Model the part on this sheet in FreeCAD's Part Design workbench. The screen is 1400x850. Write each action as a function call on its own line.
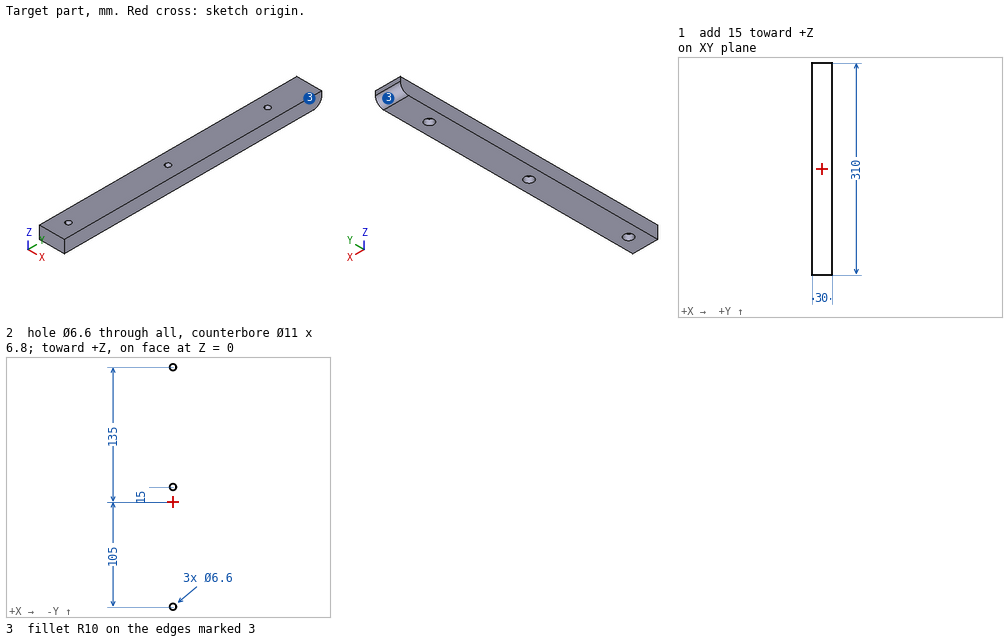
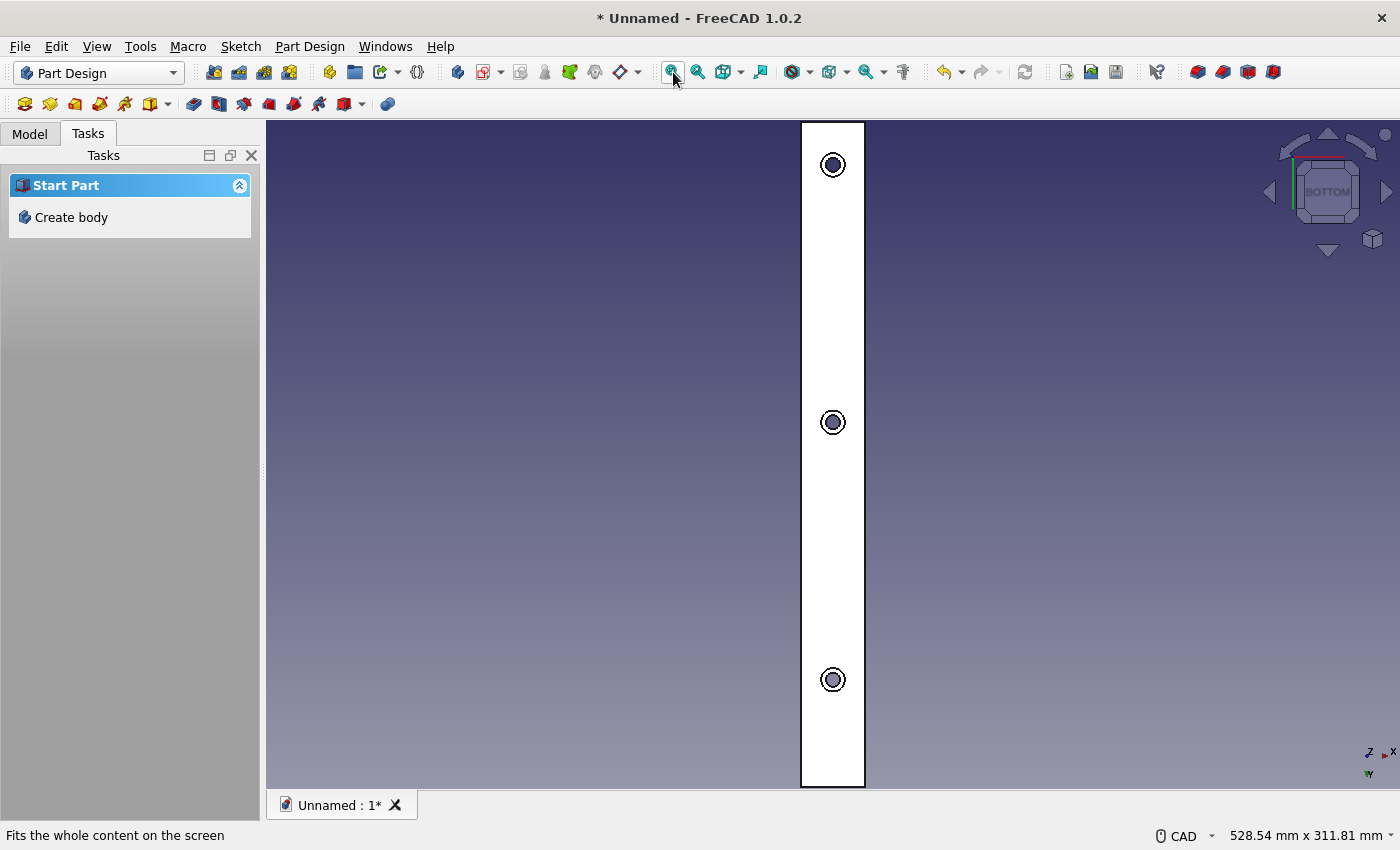
key(4)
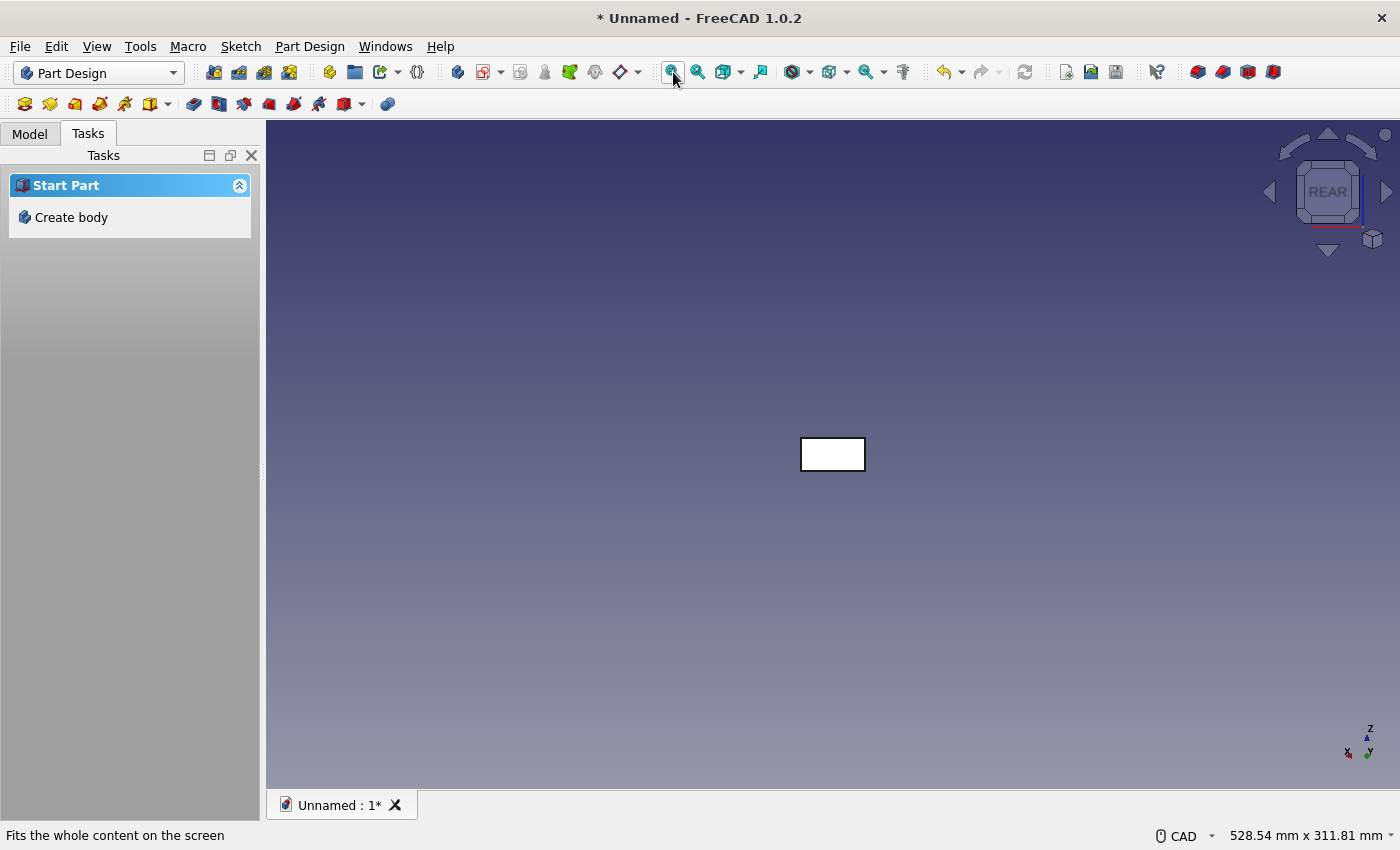
click(673, 72)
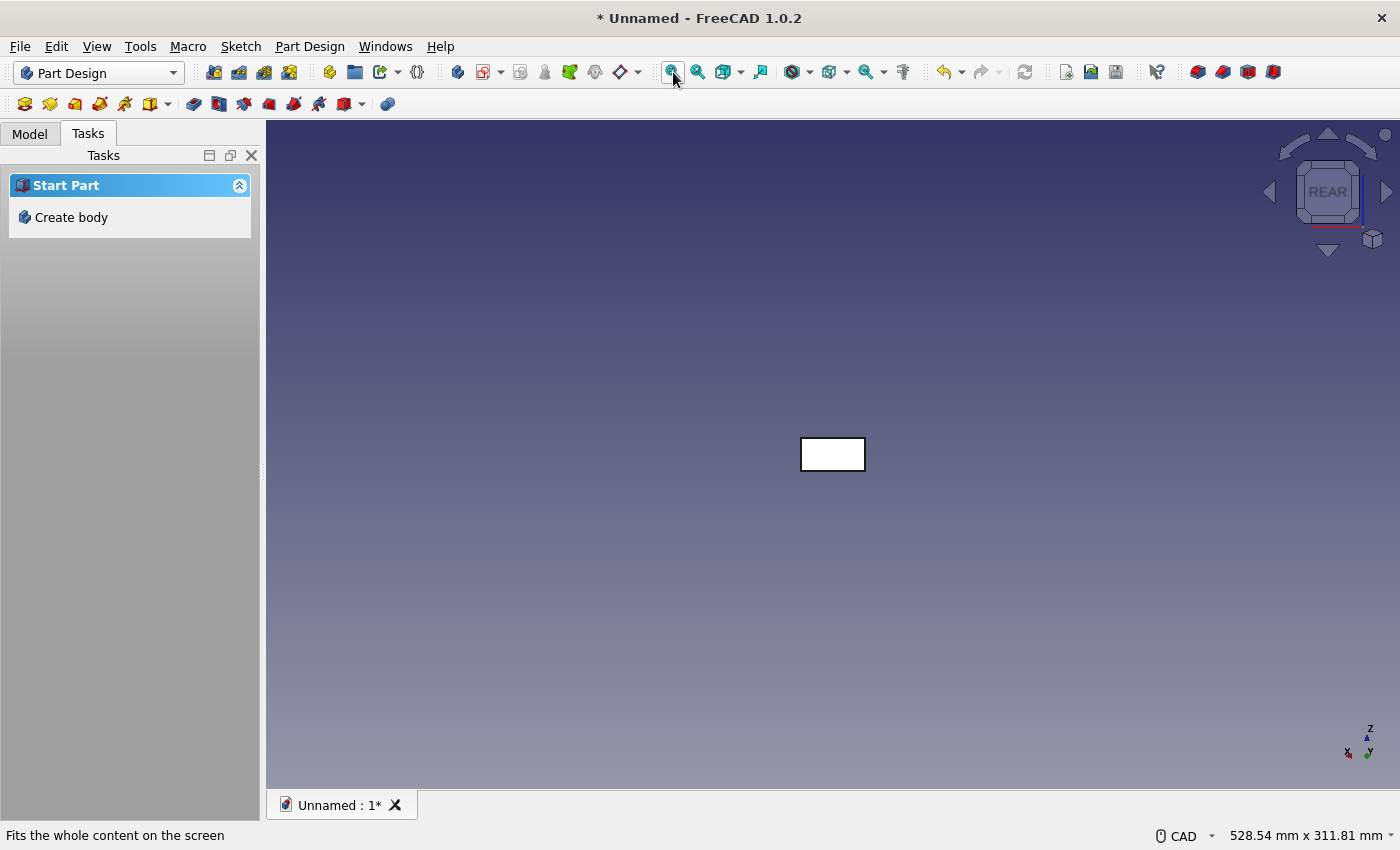
click(833, 470)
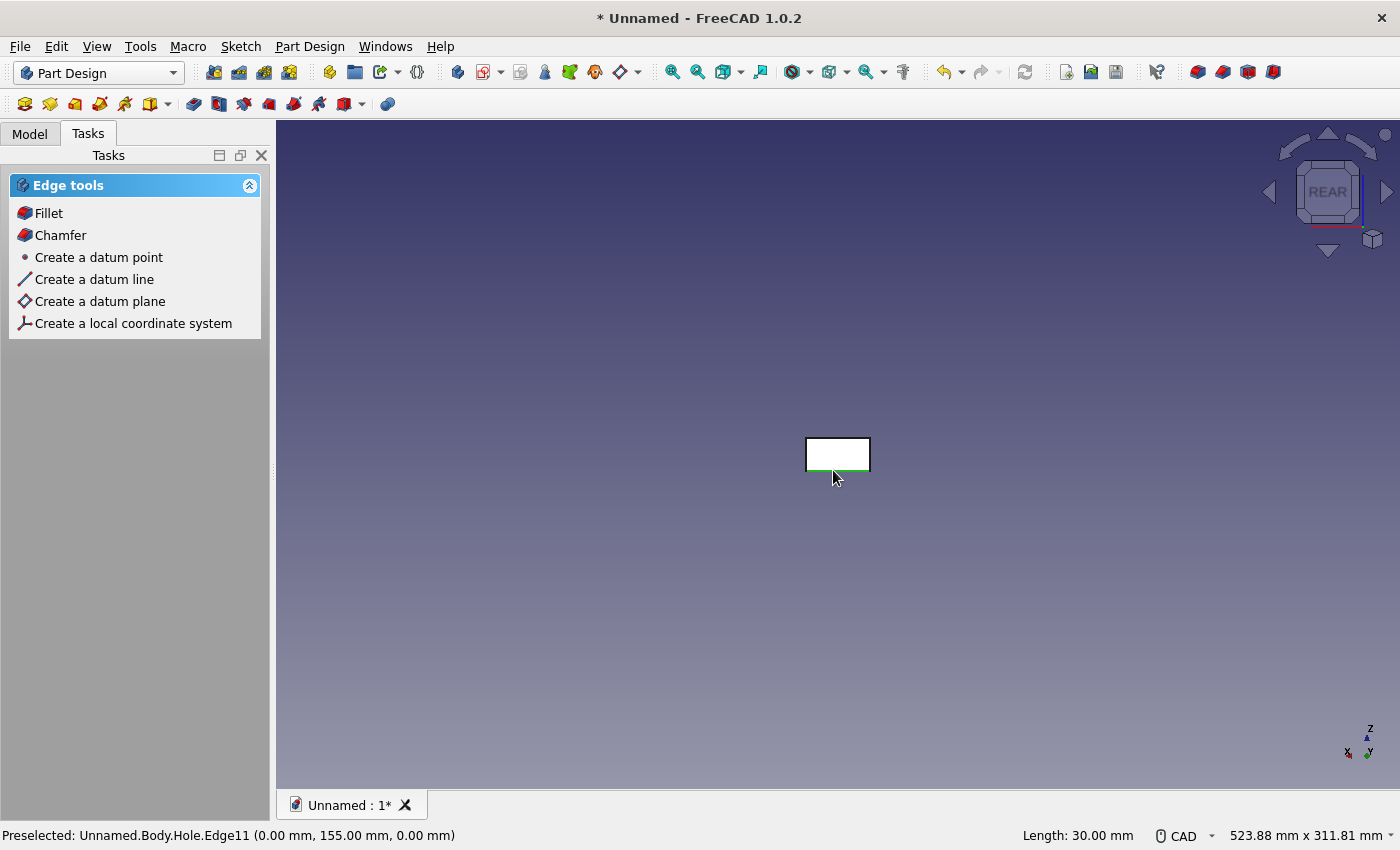
click(1198, 72)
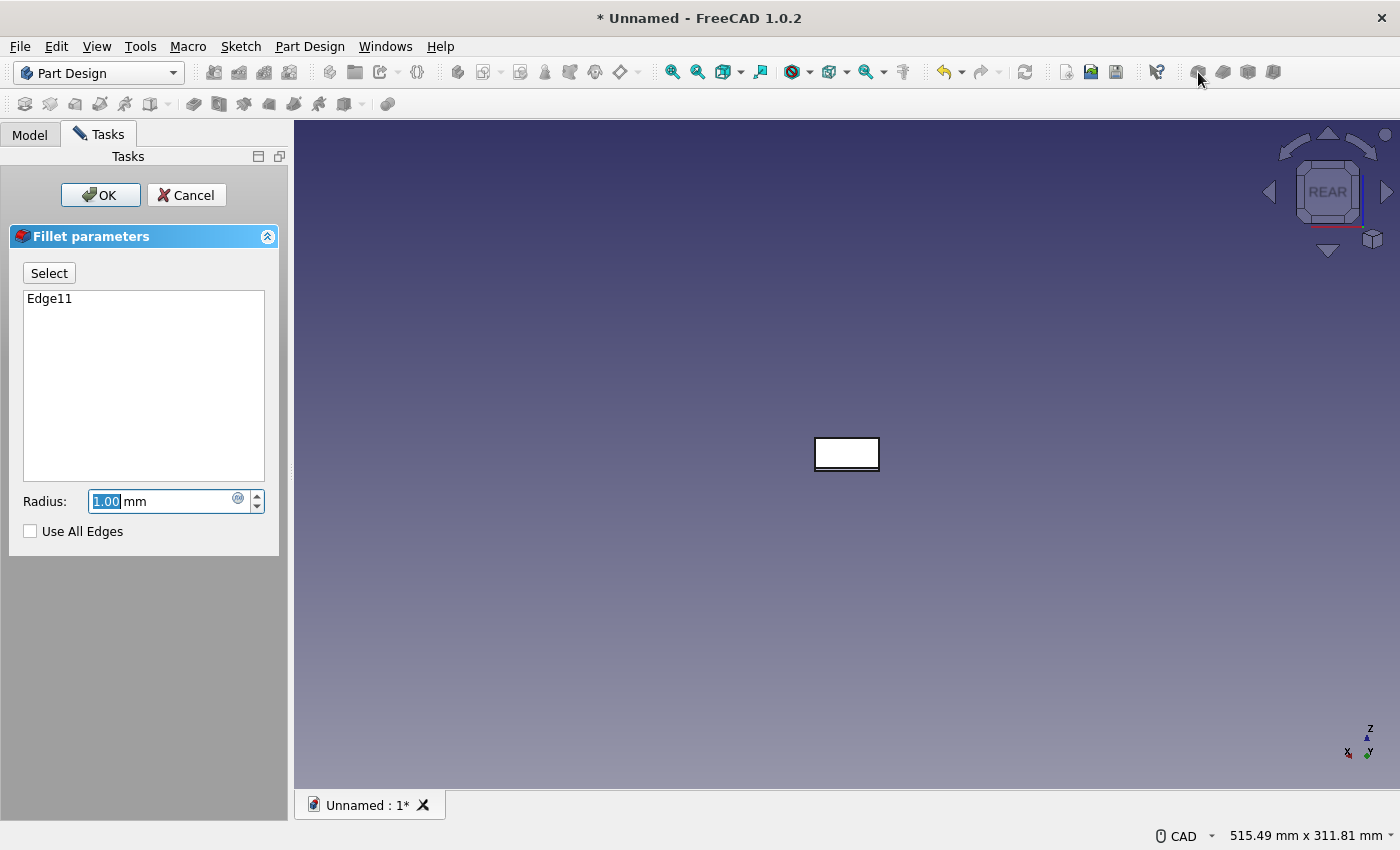
text(10)
key(Tab)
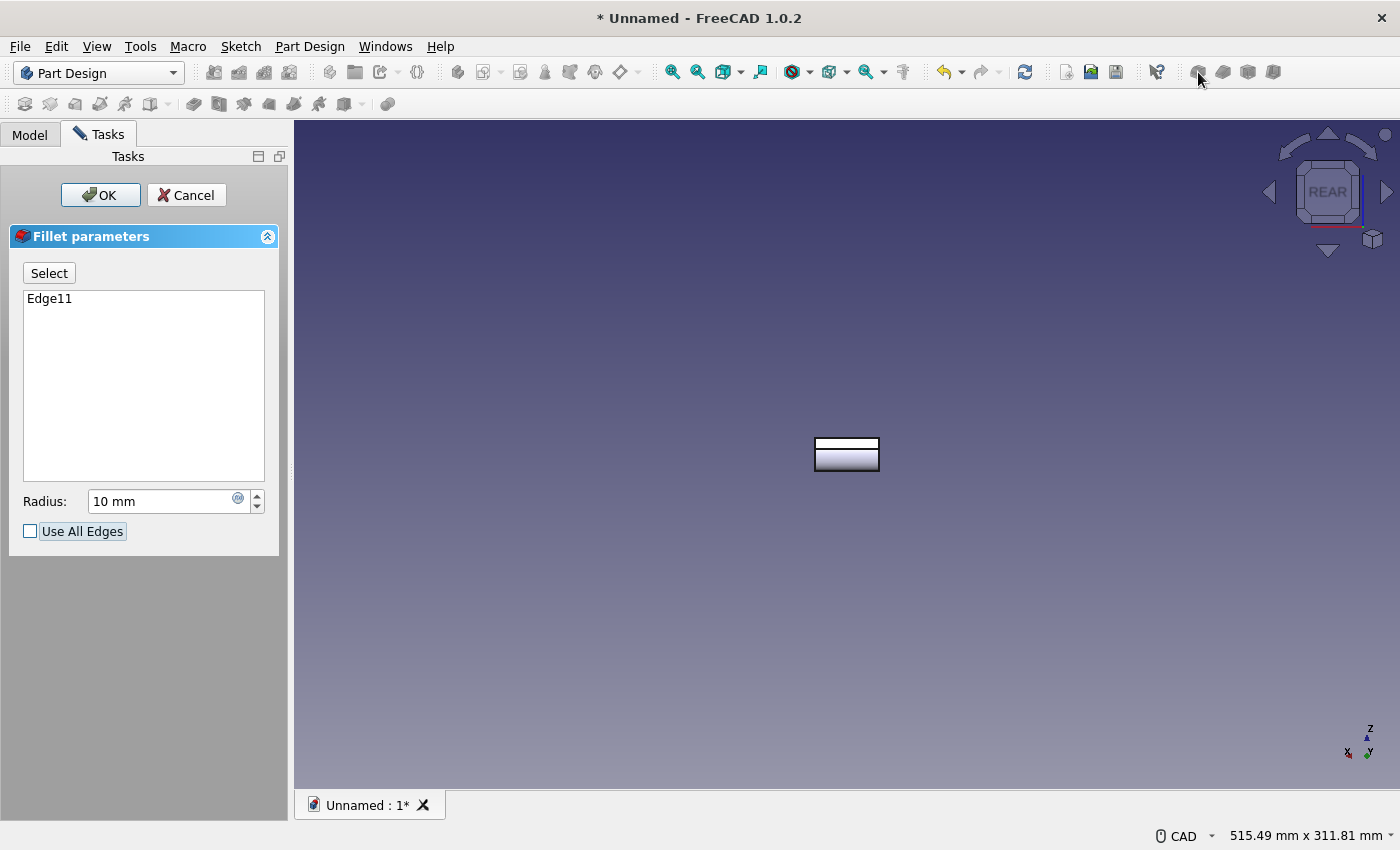
click(101, 195)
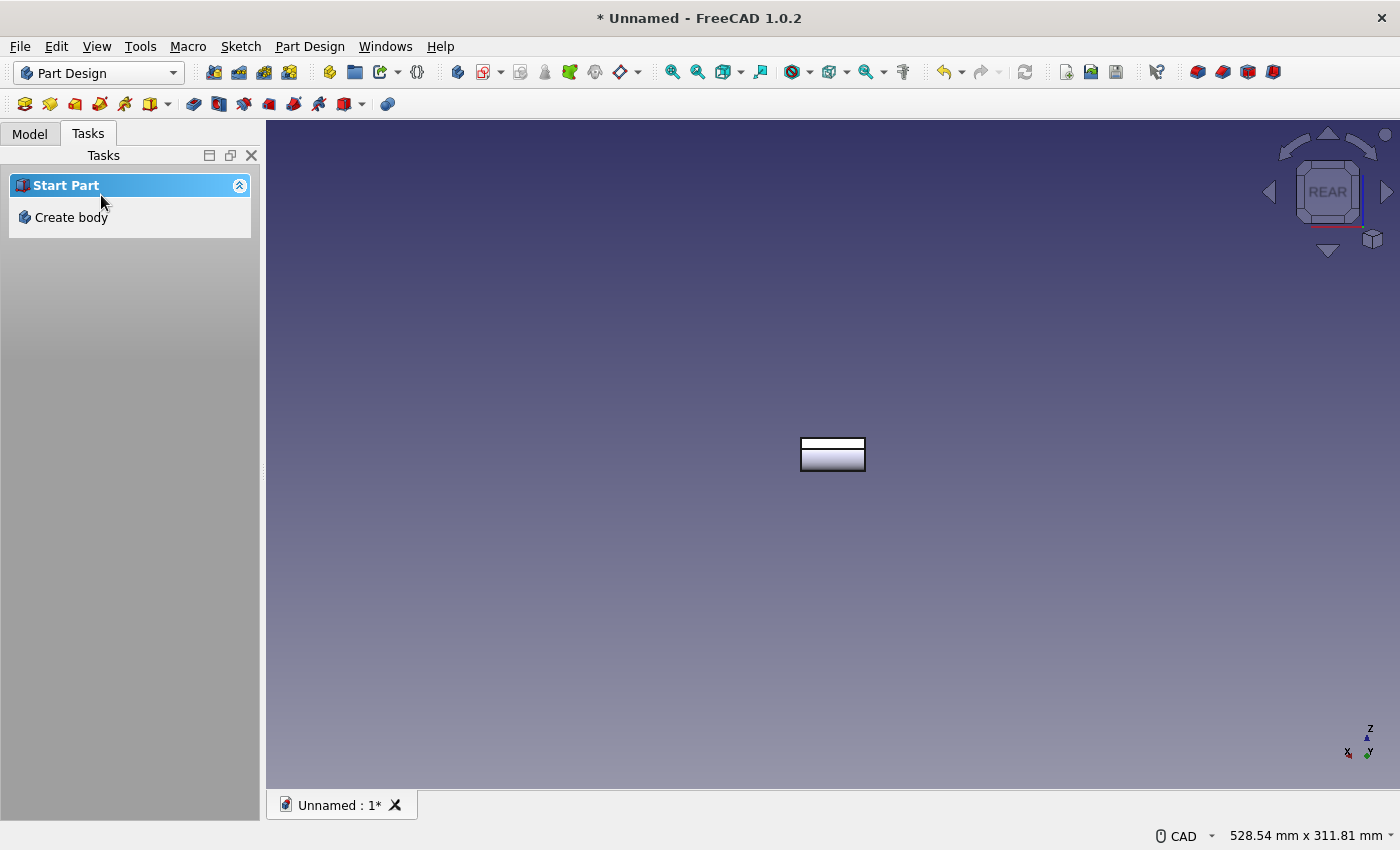
key(0)